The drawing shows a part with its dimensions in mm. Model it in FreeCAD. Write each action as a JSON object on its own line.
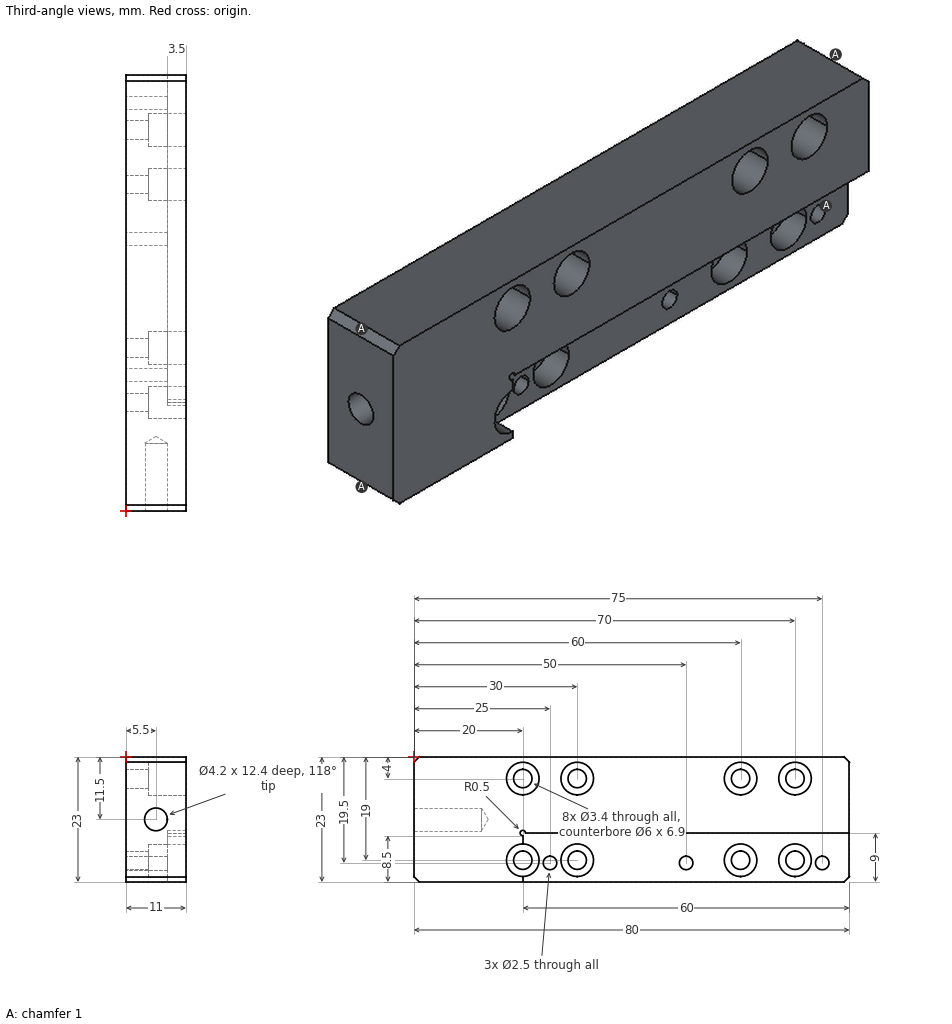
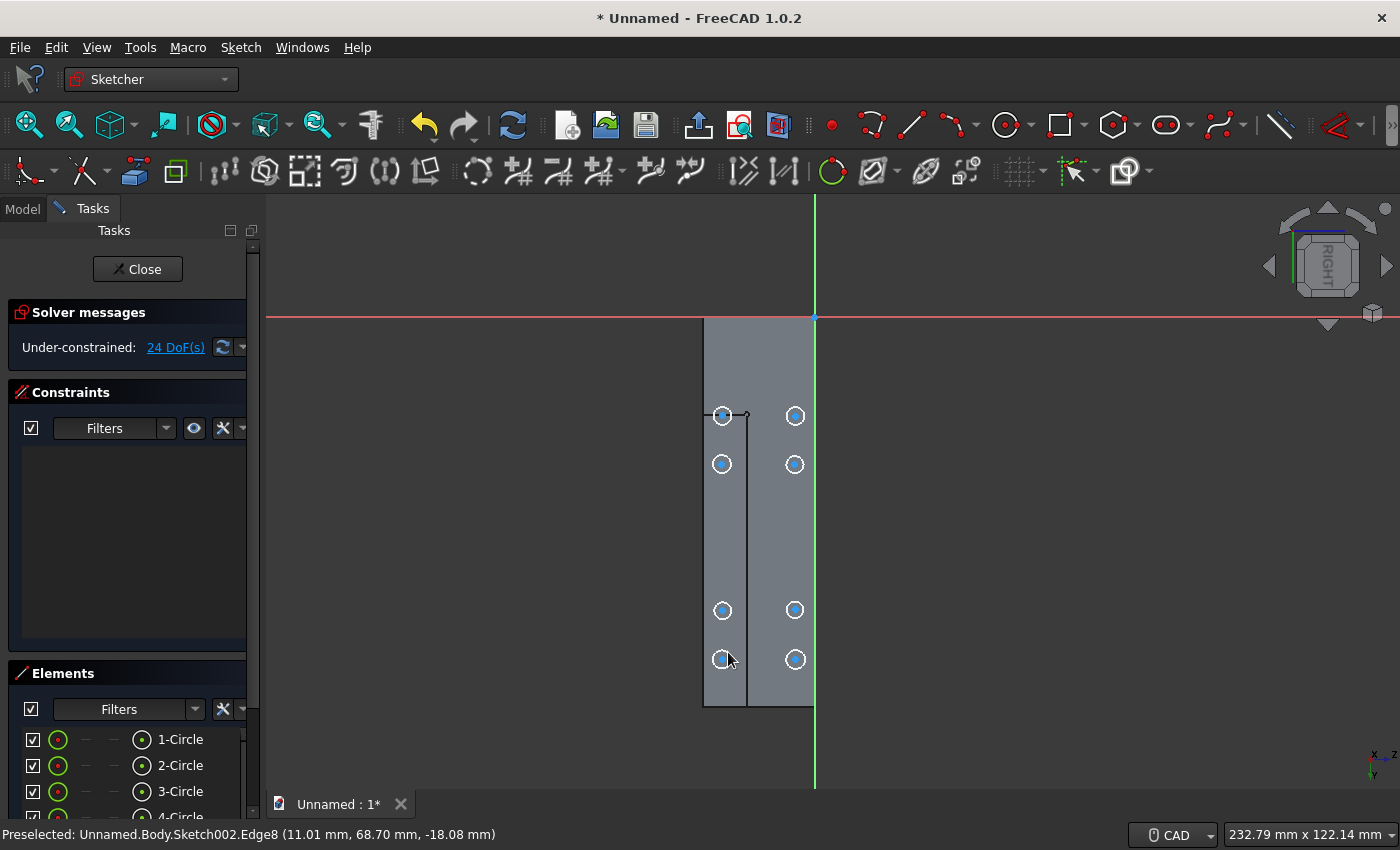
{"action": "scroll", "coordinate": [802, 410], "scroll_direction": "up", "scroll_amount": 3}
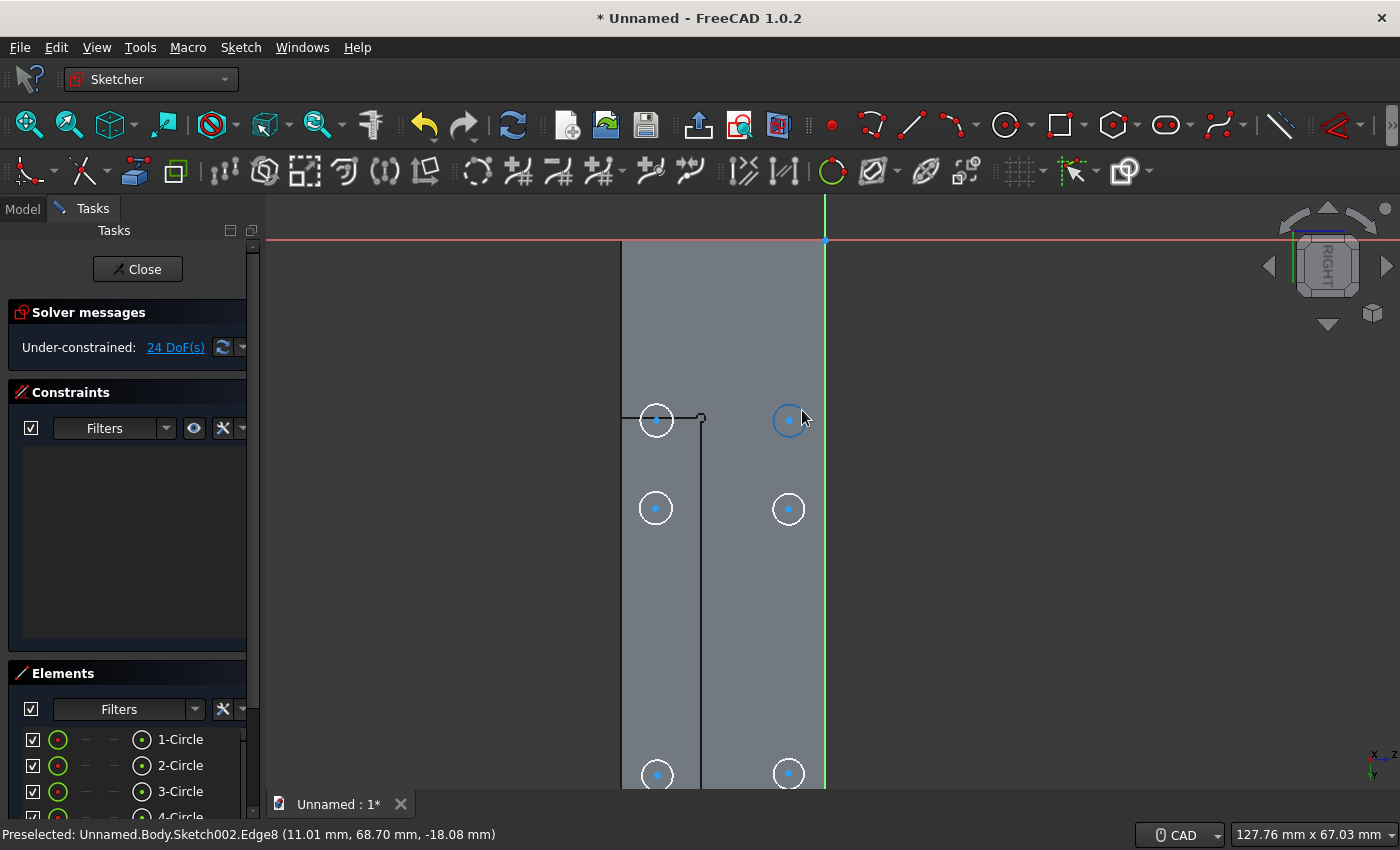
{"action": "left_click", "coordinate": [801, 409]}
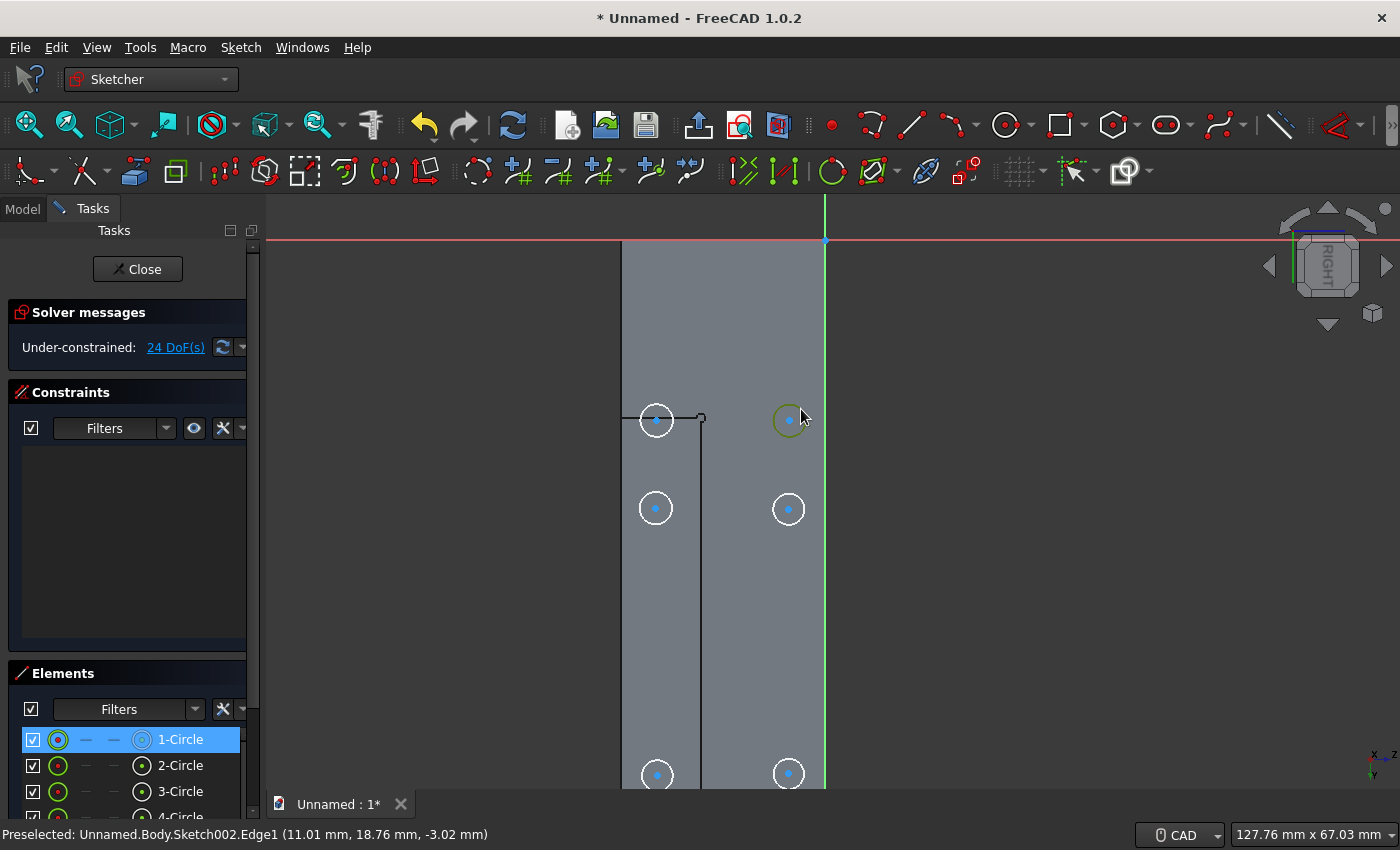
{"action": "left_click", "coordinate": [800, 498]}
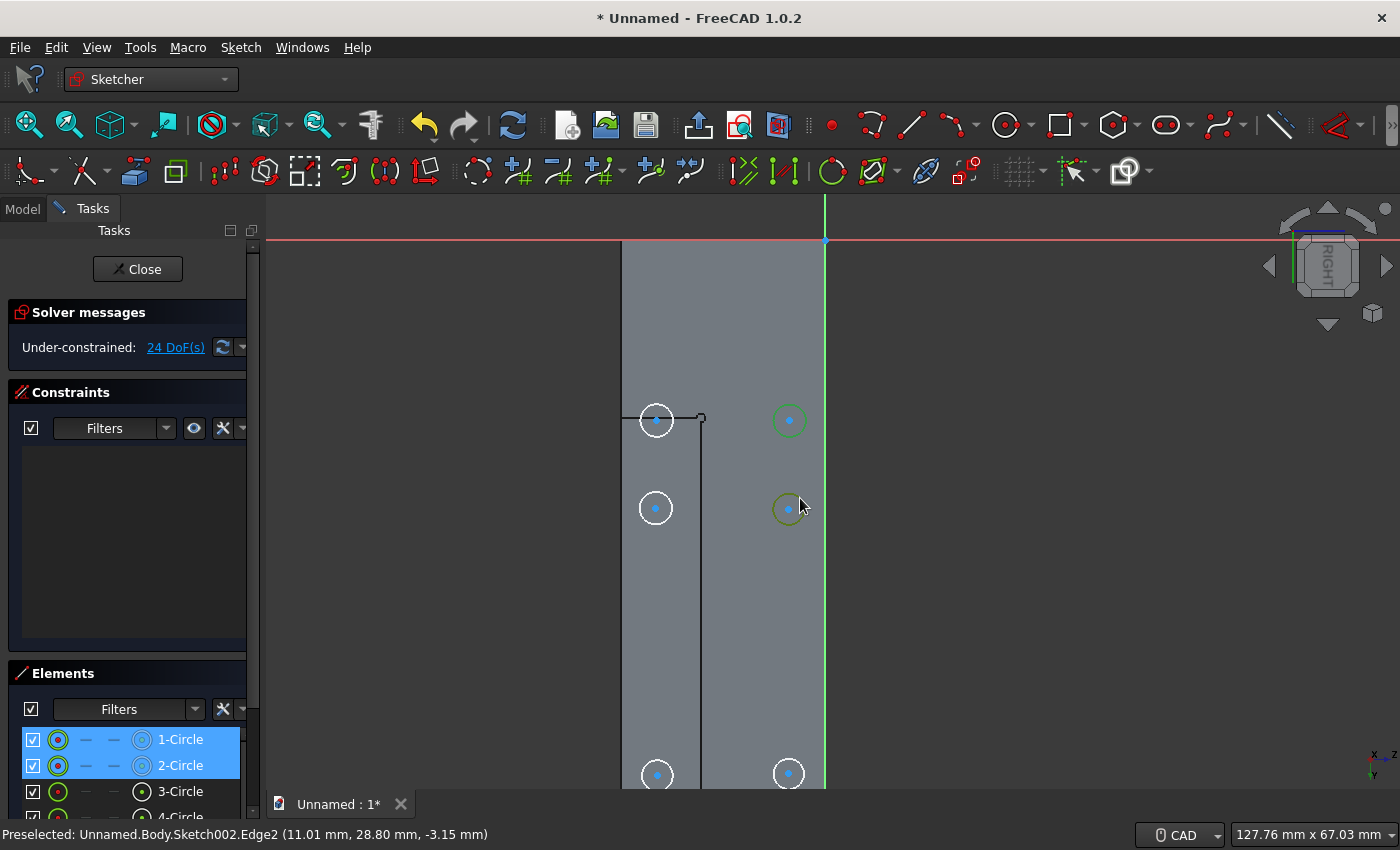
{"action": "left_click", "coordinate": [667, 497]}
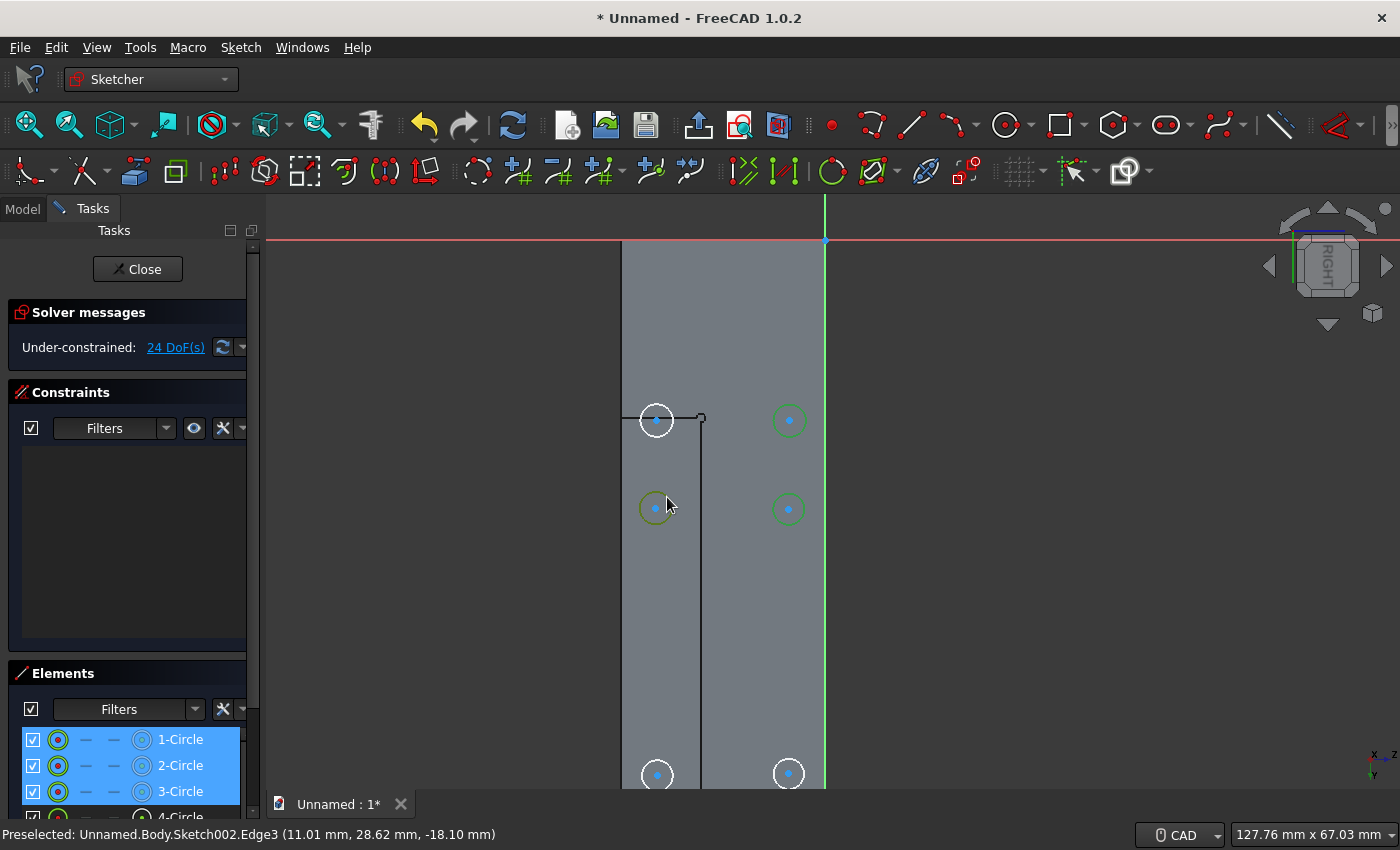
{"action": "left_click", "coordinate": [668, 409]}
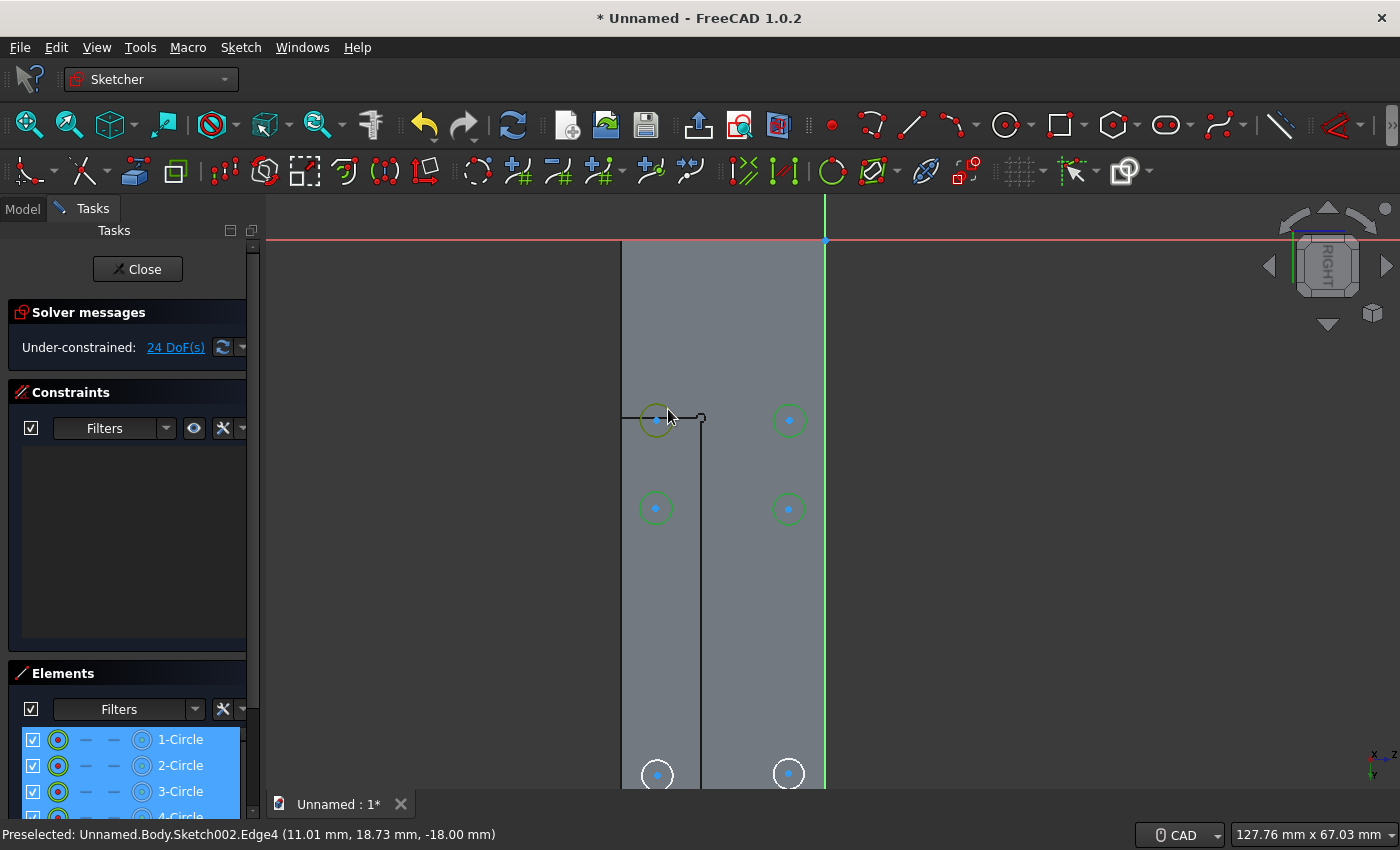
{"action": "left_click", "coordinate": [789, 759]}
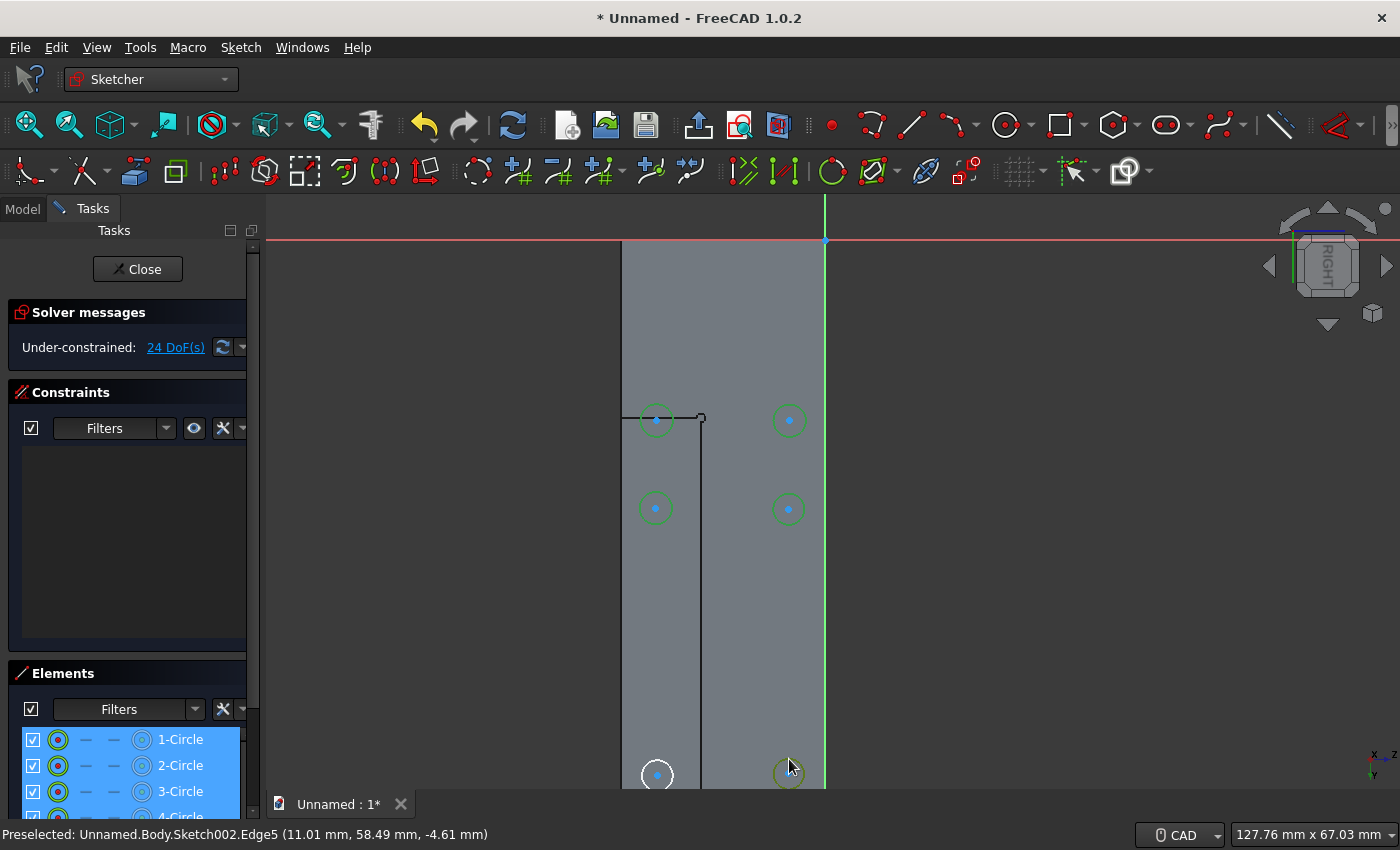
{"action": "scroll", "coordinate": [802, 410], "scroll_direction": "down", "scroll_amount": 3}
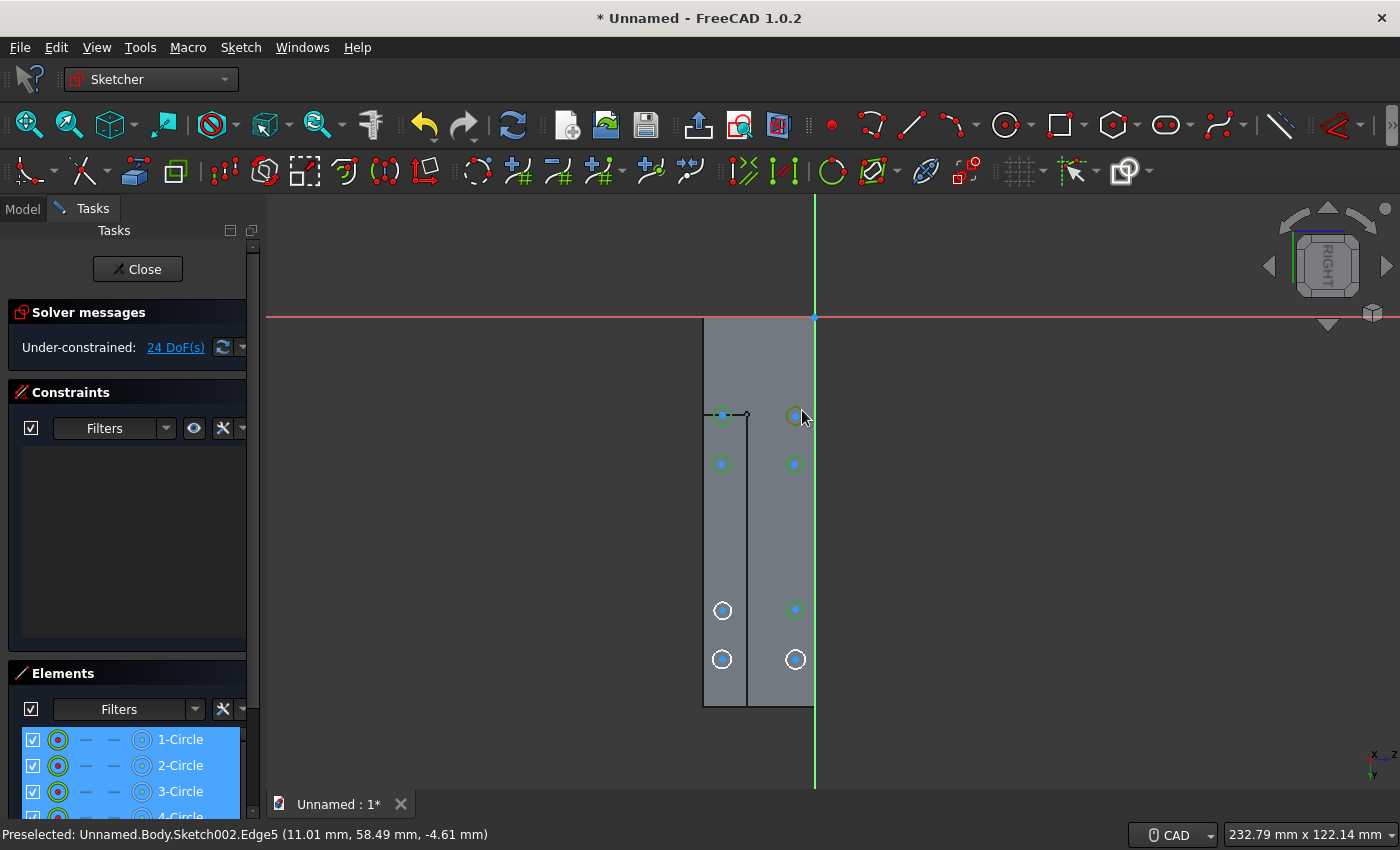
{"action": "scroll", "coordinate": [802, 653], "scroll_direction": "up", "scroll_amount": 2}